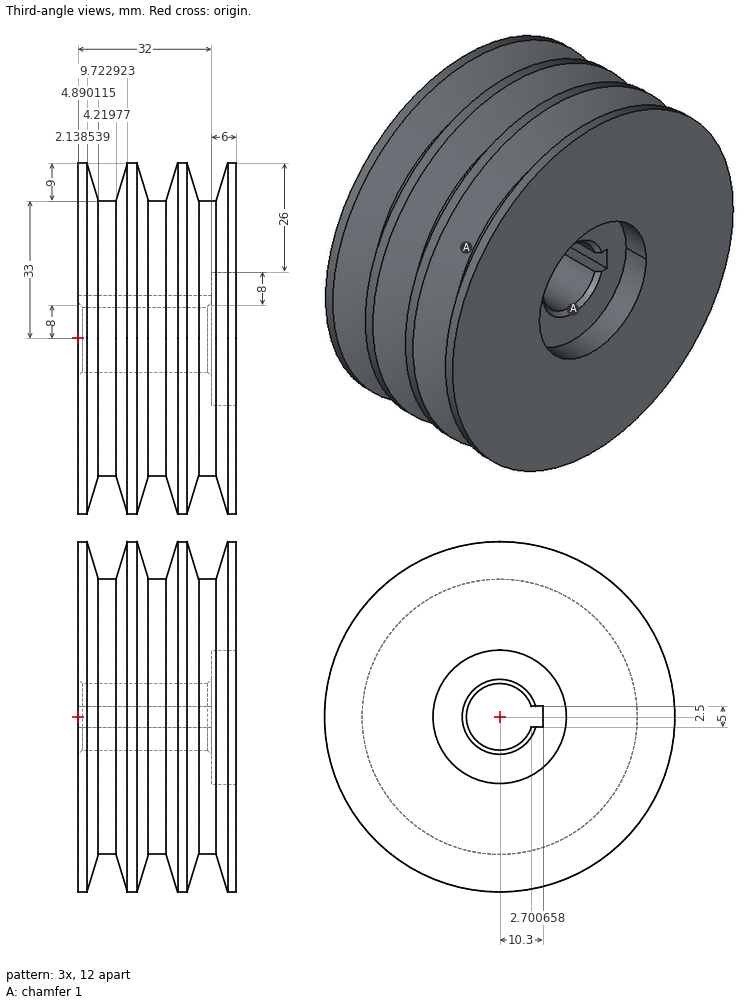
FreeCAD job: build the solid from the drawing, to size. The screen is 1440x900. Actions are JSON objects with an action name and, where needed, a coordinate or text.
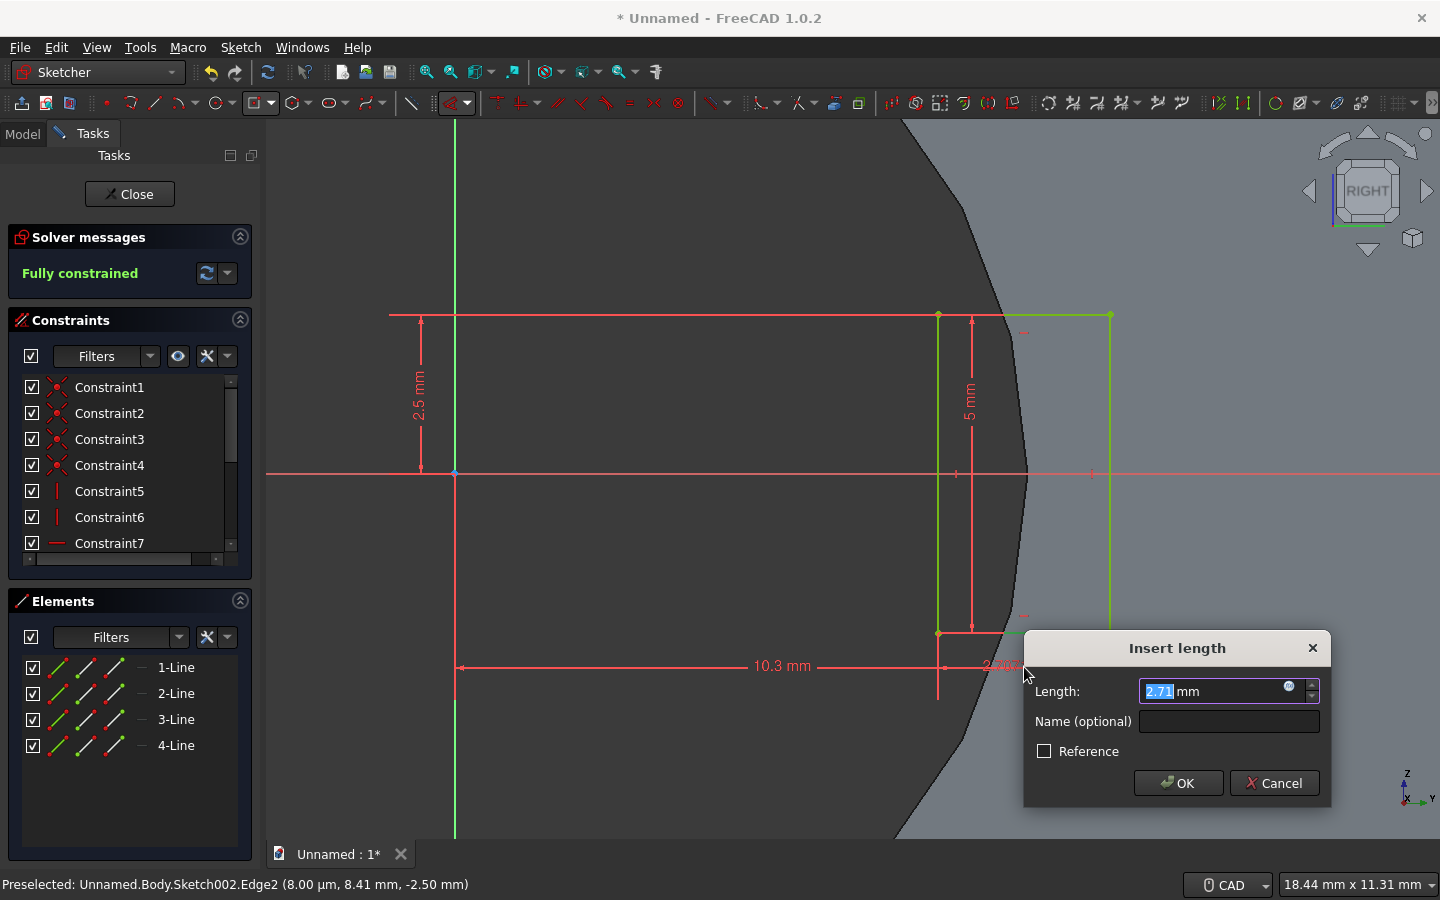
{"action": "type", "text": "2.700658"}
{"action": "key", "text": "Return"}
{"action": "key", "text": "Escape"}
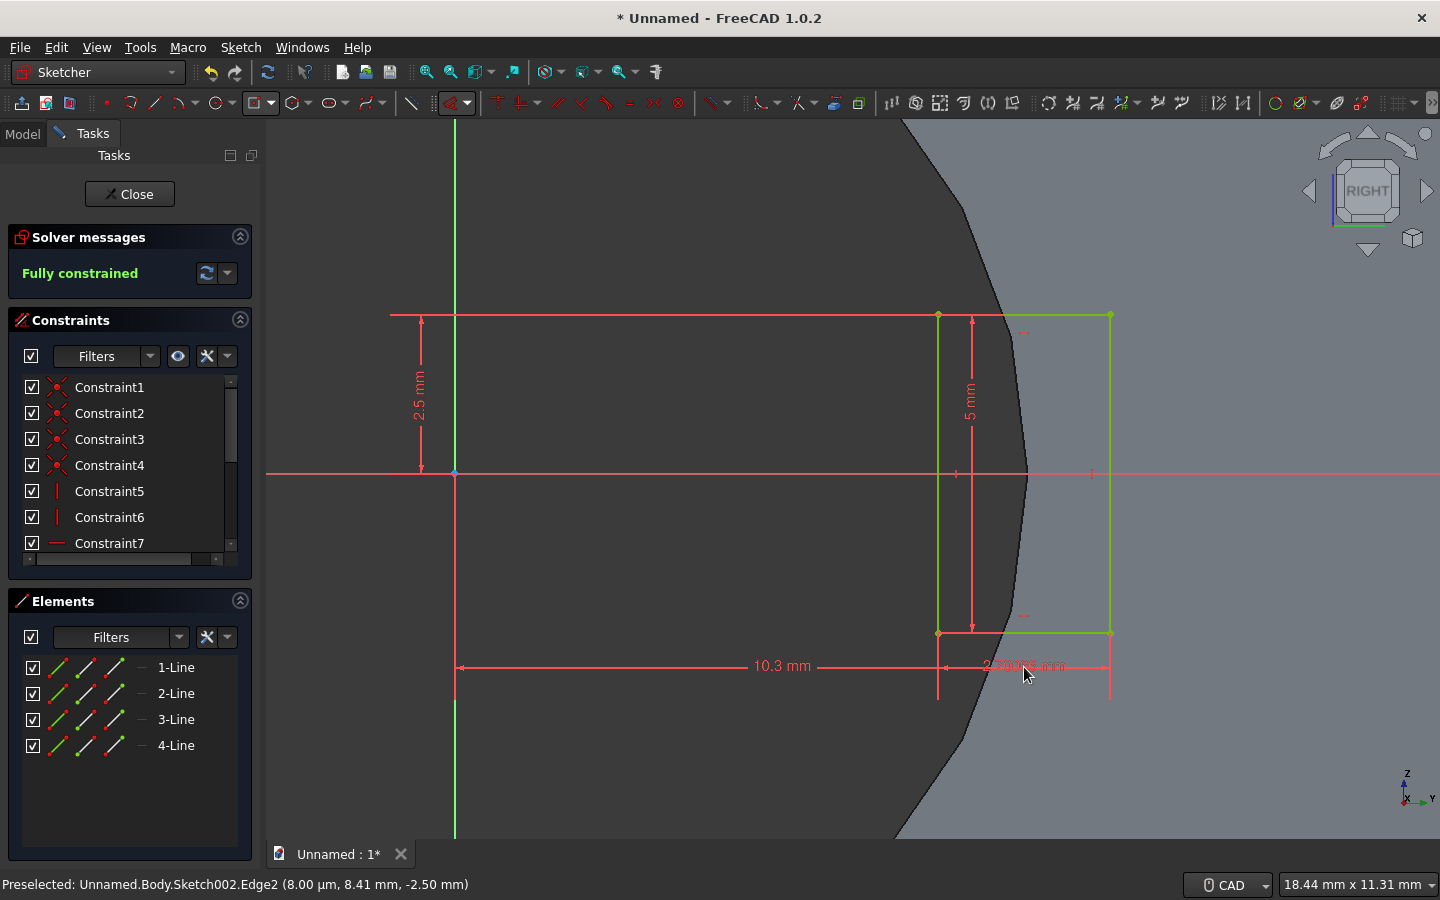
{"action": "left_click", "coordinate": [130, 194]}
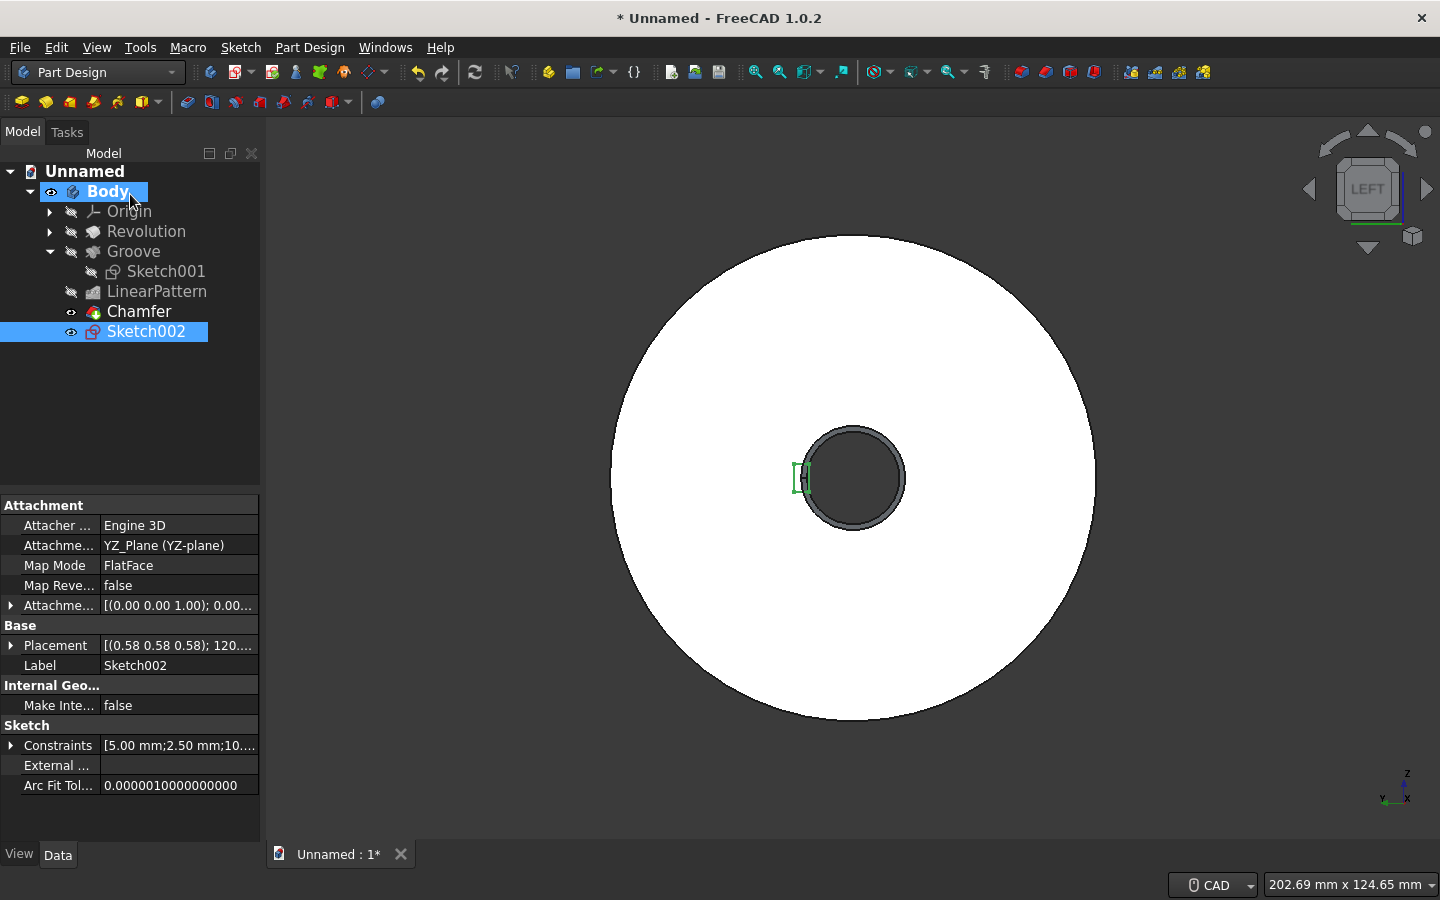
{"action": "left_click", "coordinate": [188, 102]}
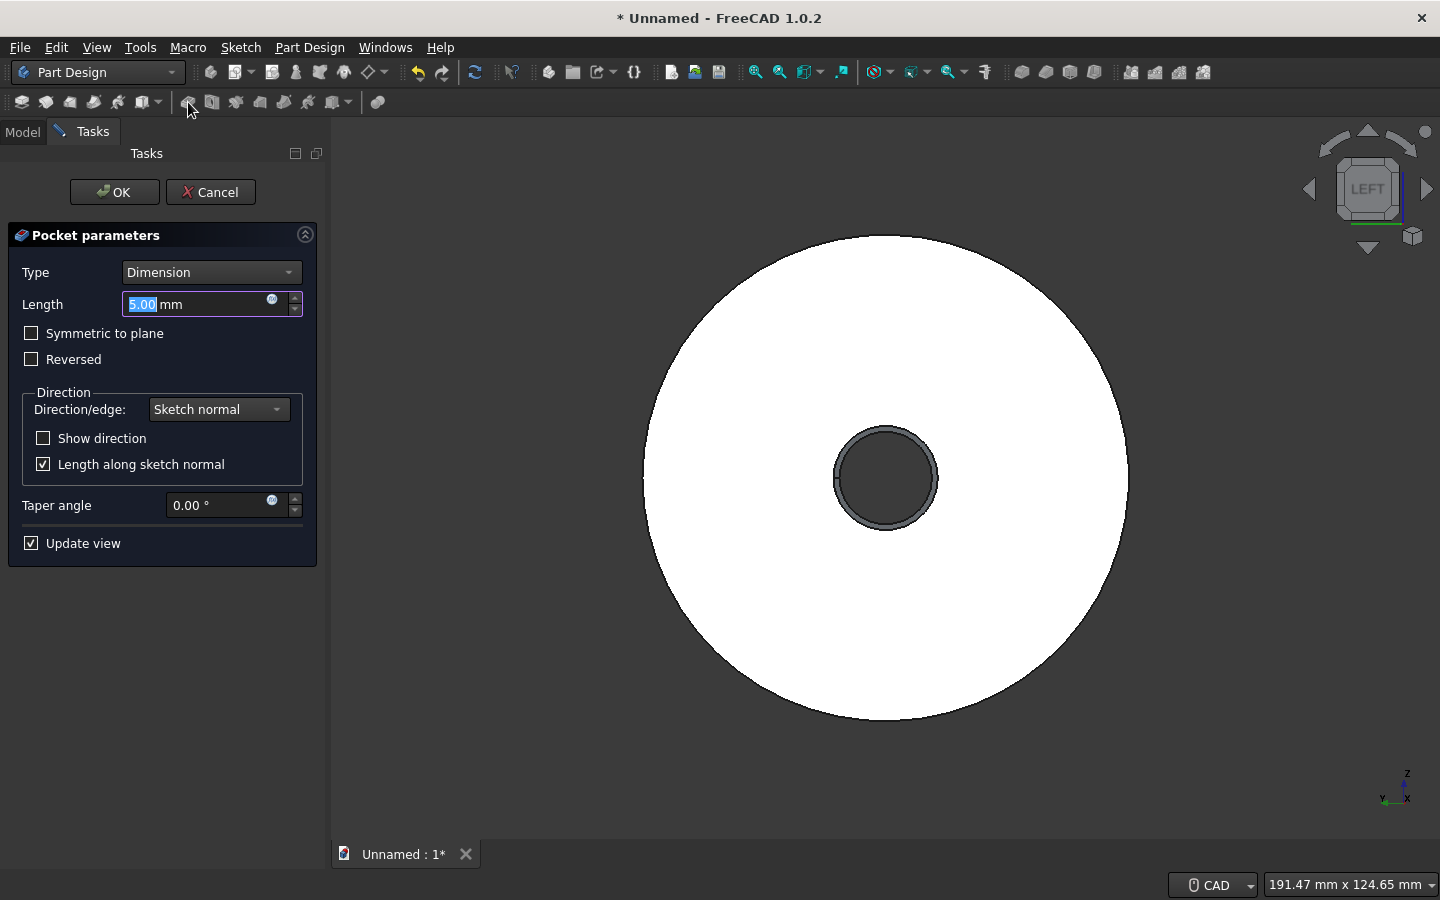
{"action": "left_click", "coordinate": [212, 272]}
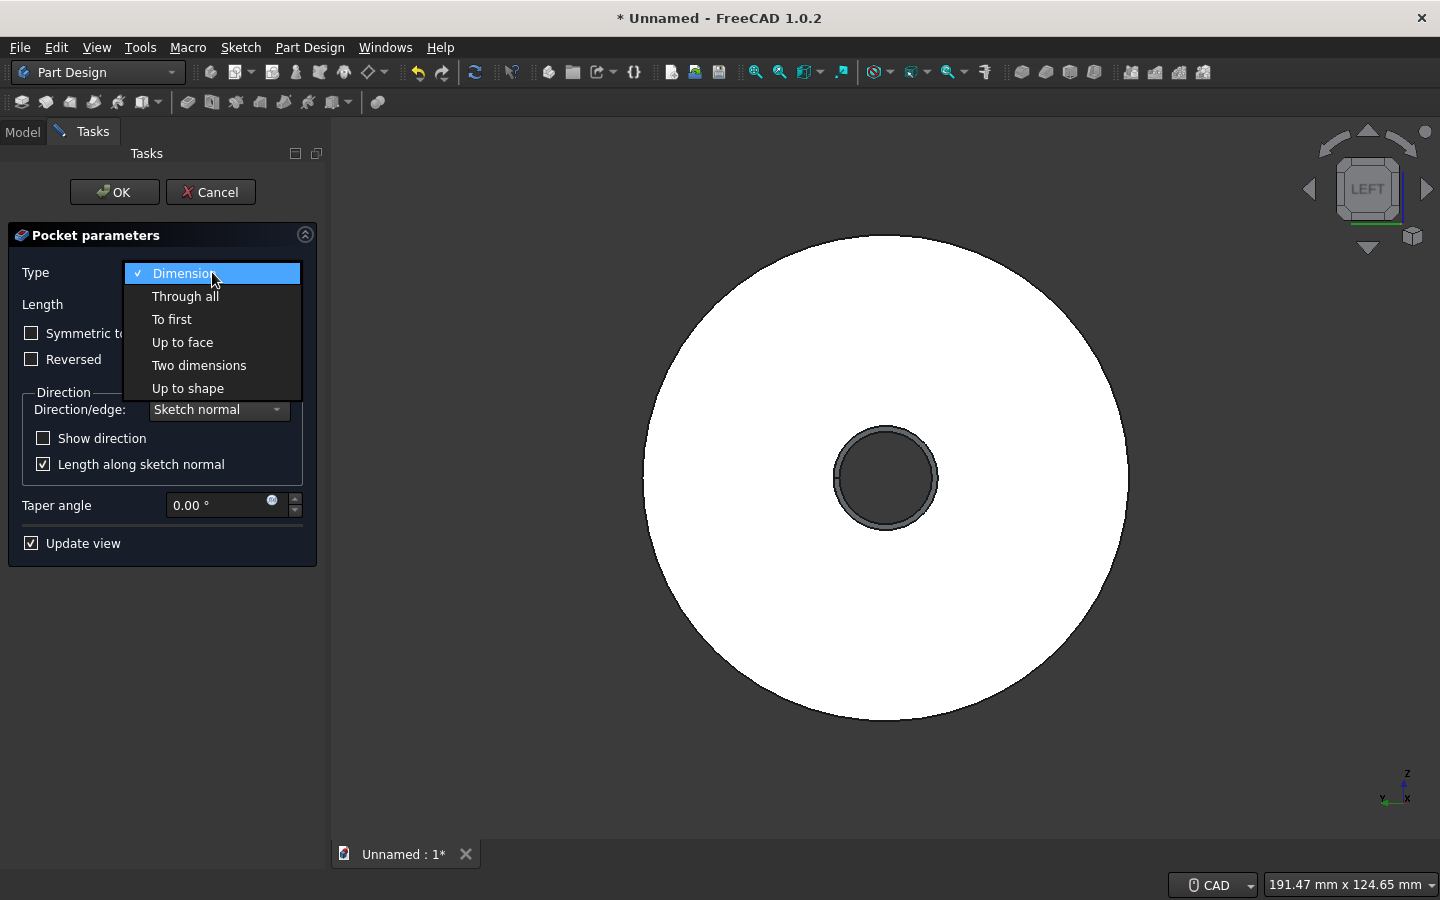
{"action": "left_click", "coordinate": [212, 296]}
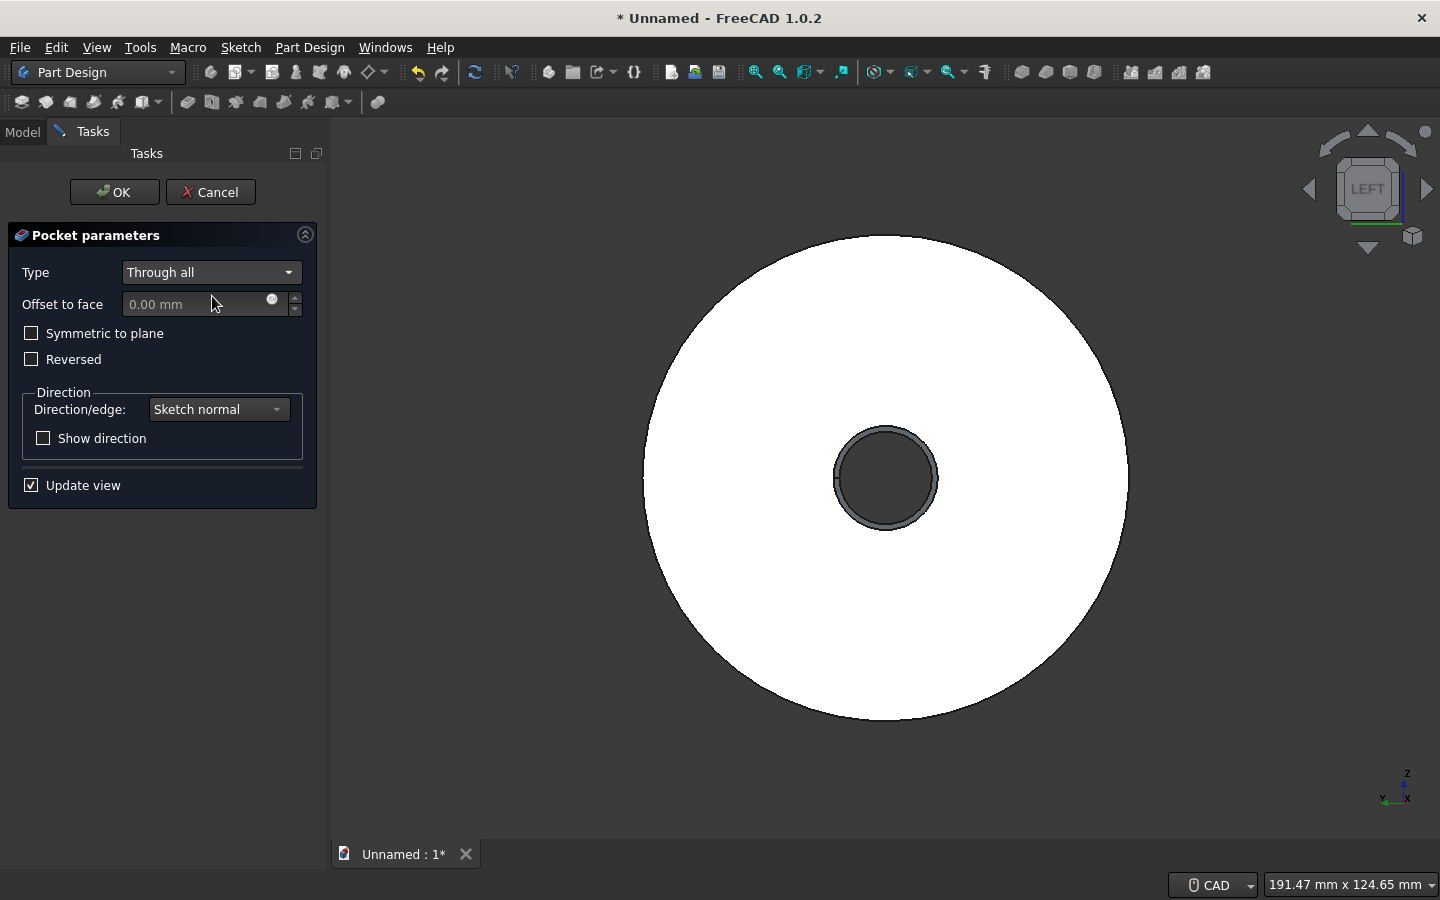
{"action": "left_click", "coordinate": [30, 359]}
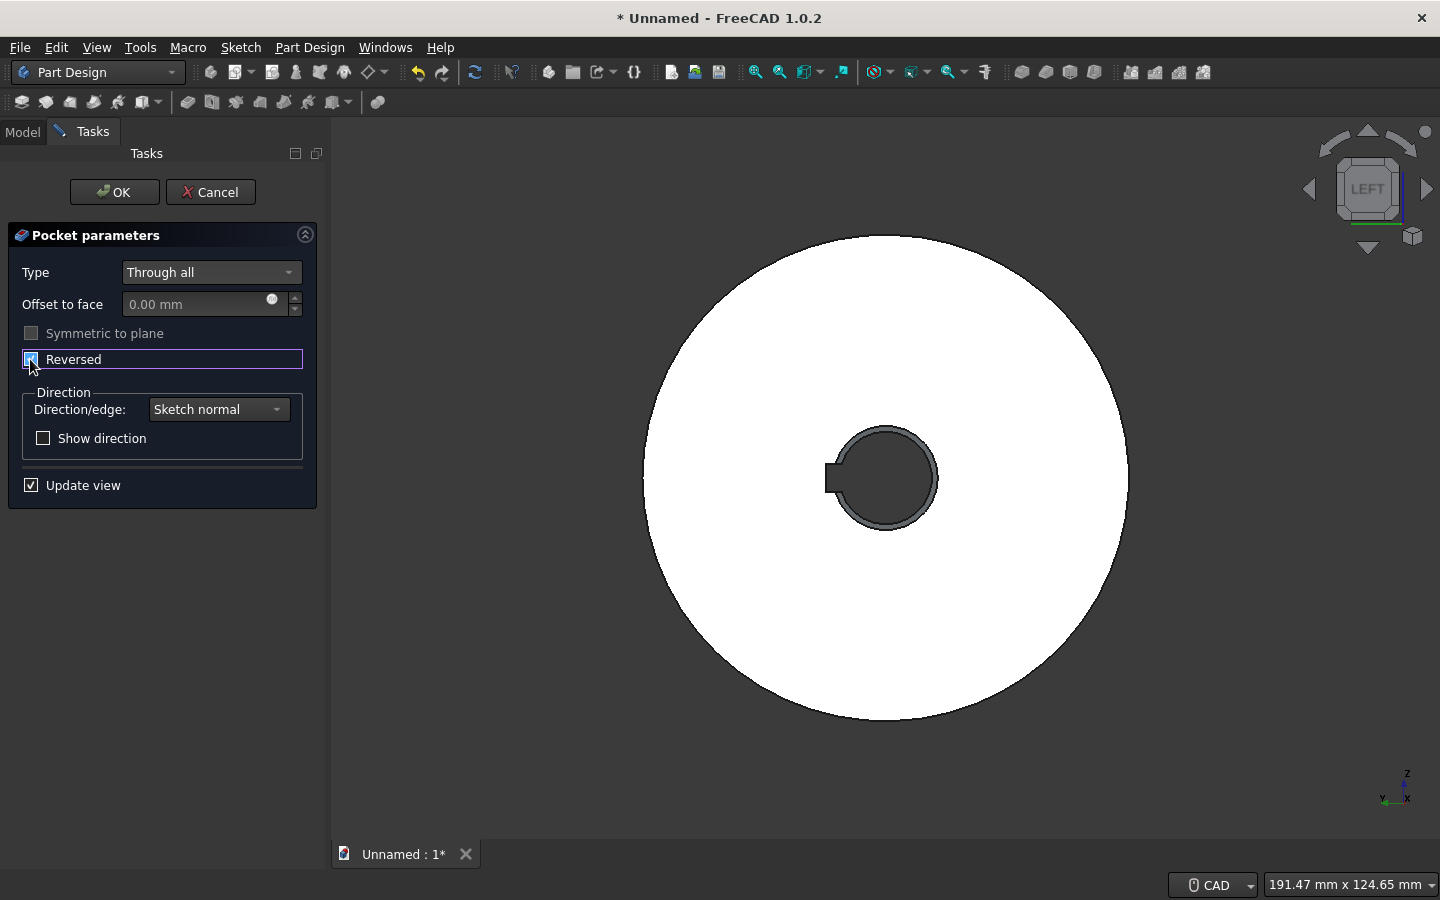
{"action": "left_click", "coordinate": [115, 192]}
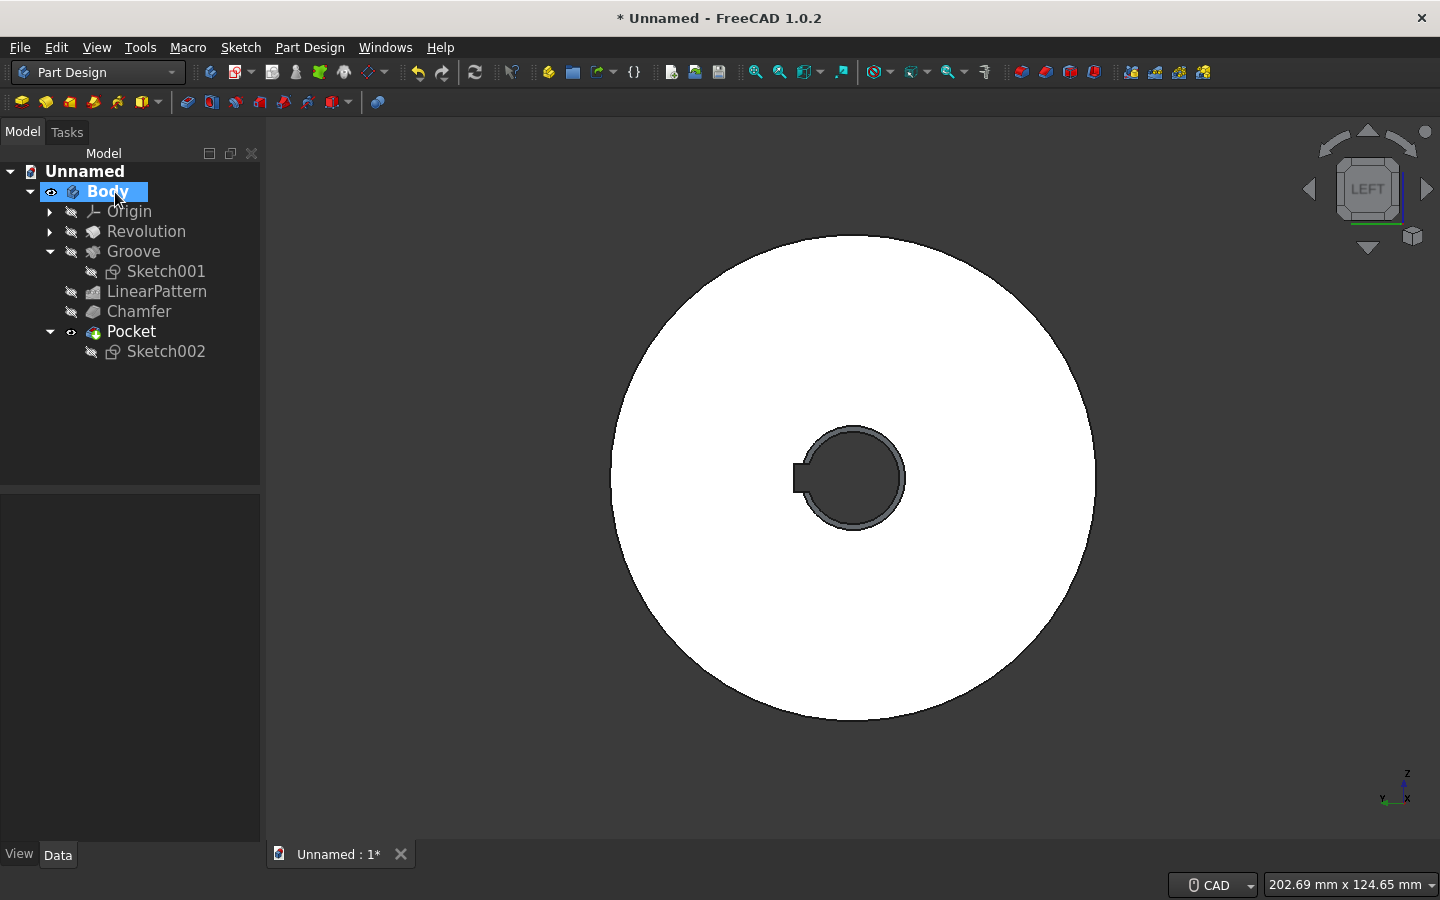
{"action": "key", "text": "0"}